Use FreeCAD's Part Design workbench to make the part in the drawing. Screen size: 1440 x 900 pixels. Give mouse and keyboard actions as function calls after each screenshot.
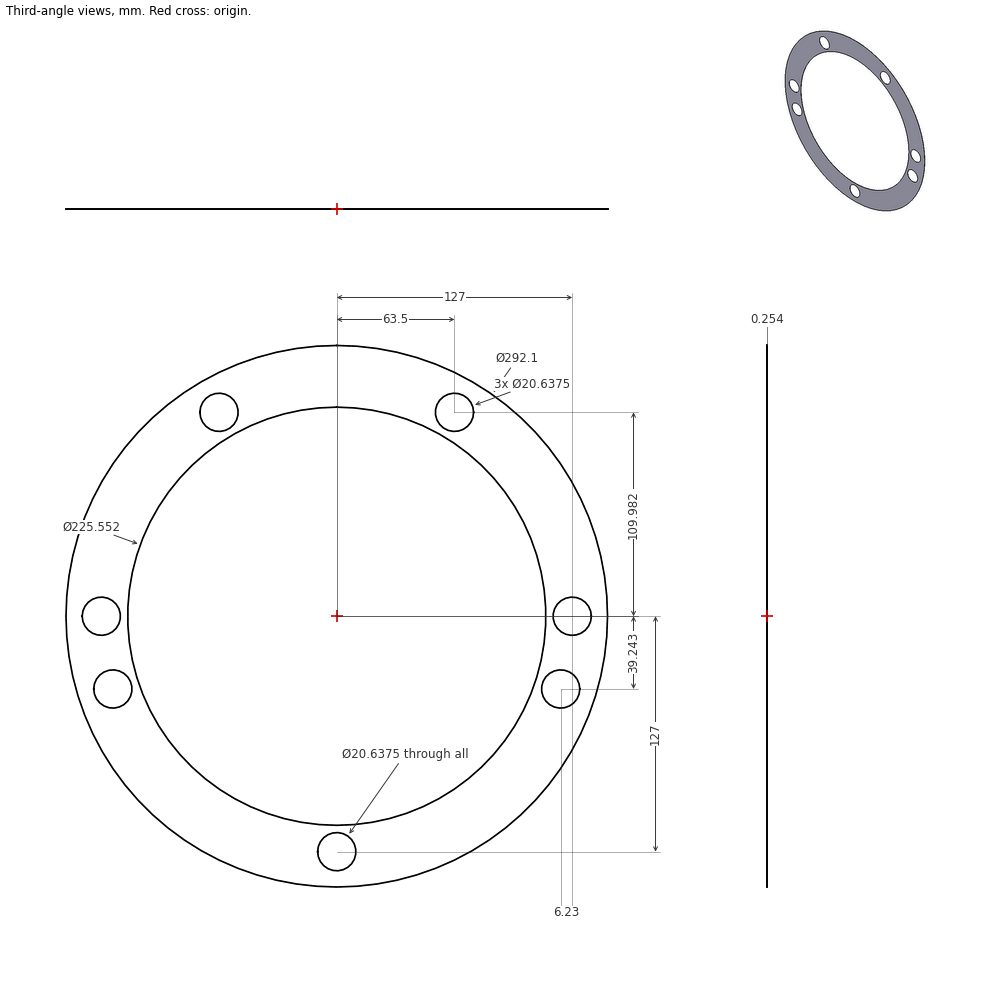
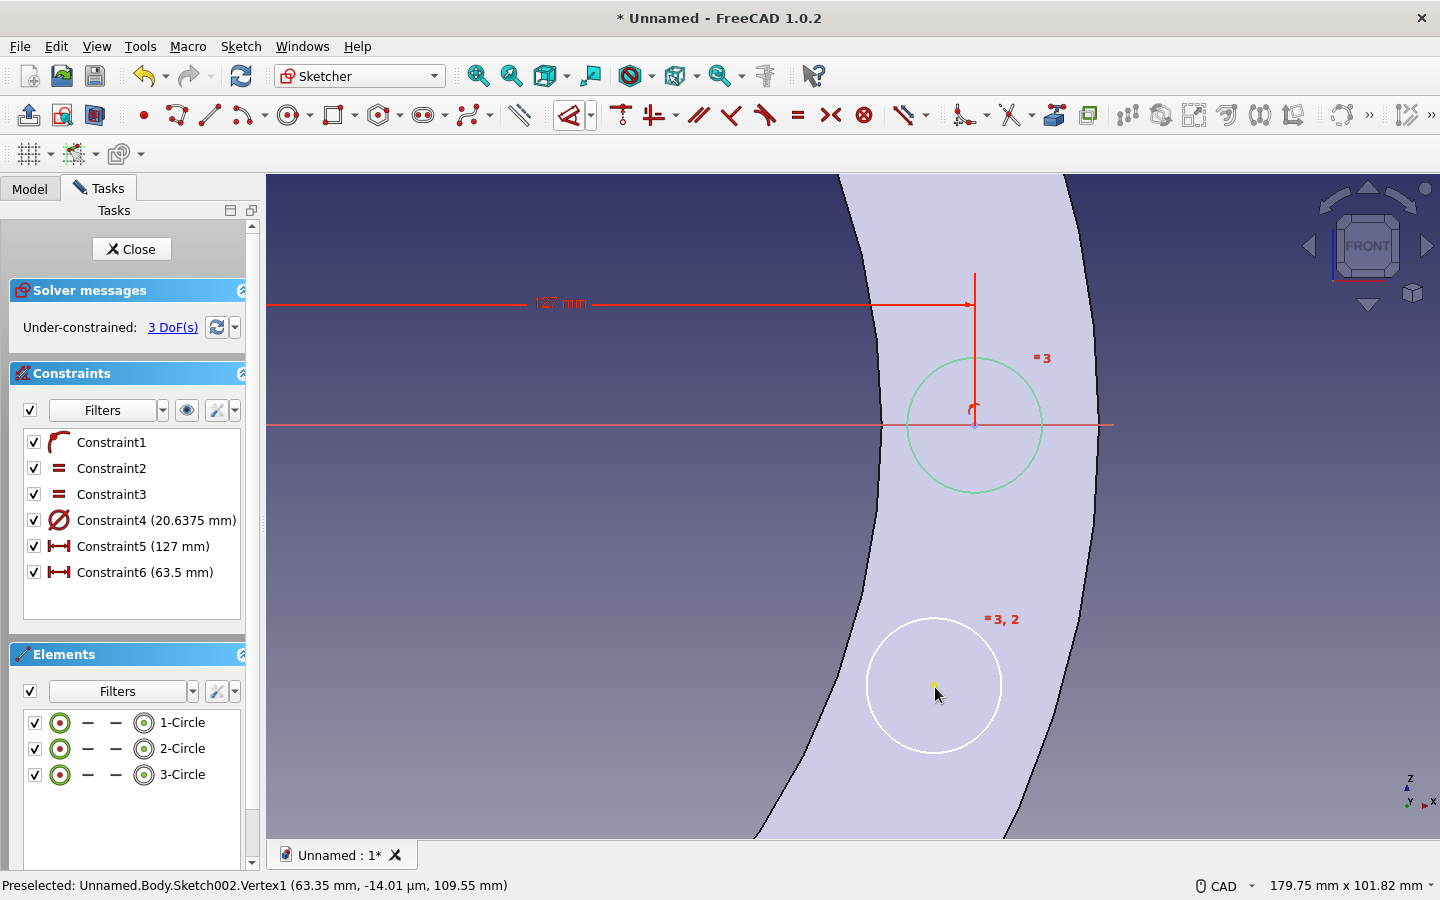
click(934, 686)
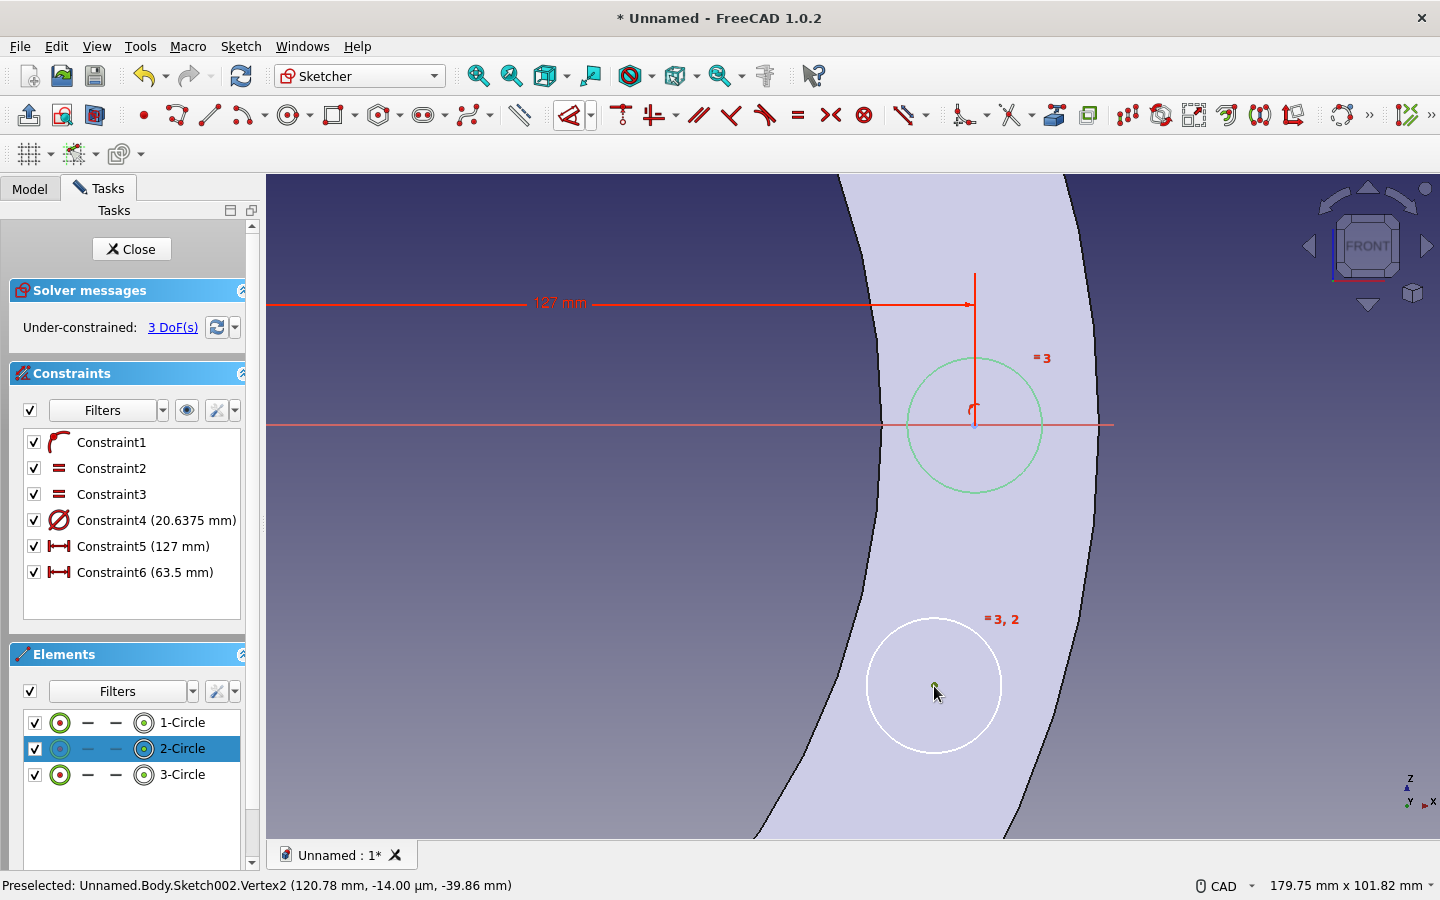
click(975, 425)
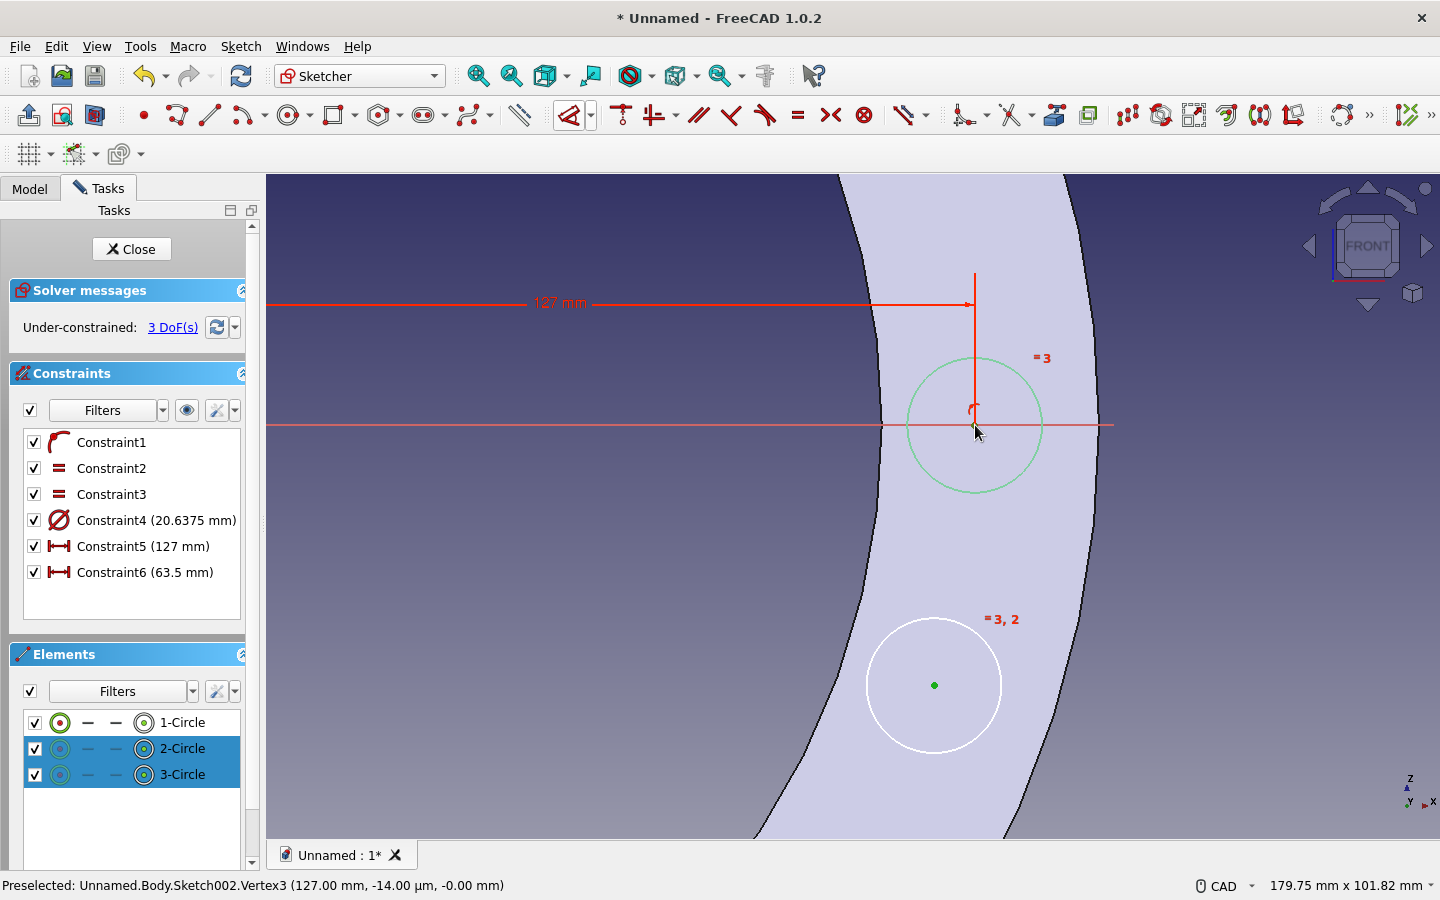
click(590, 116)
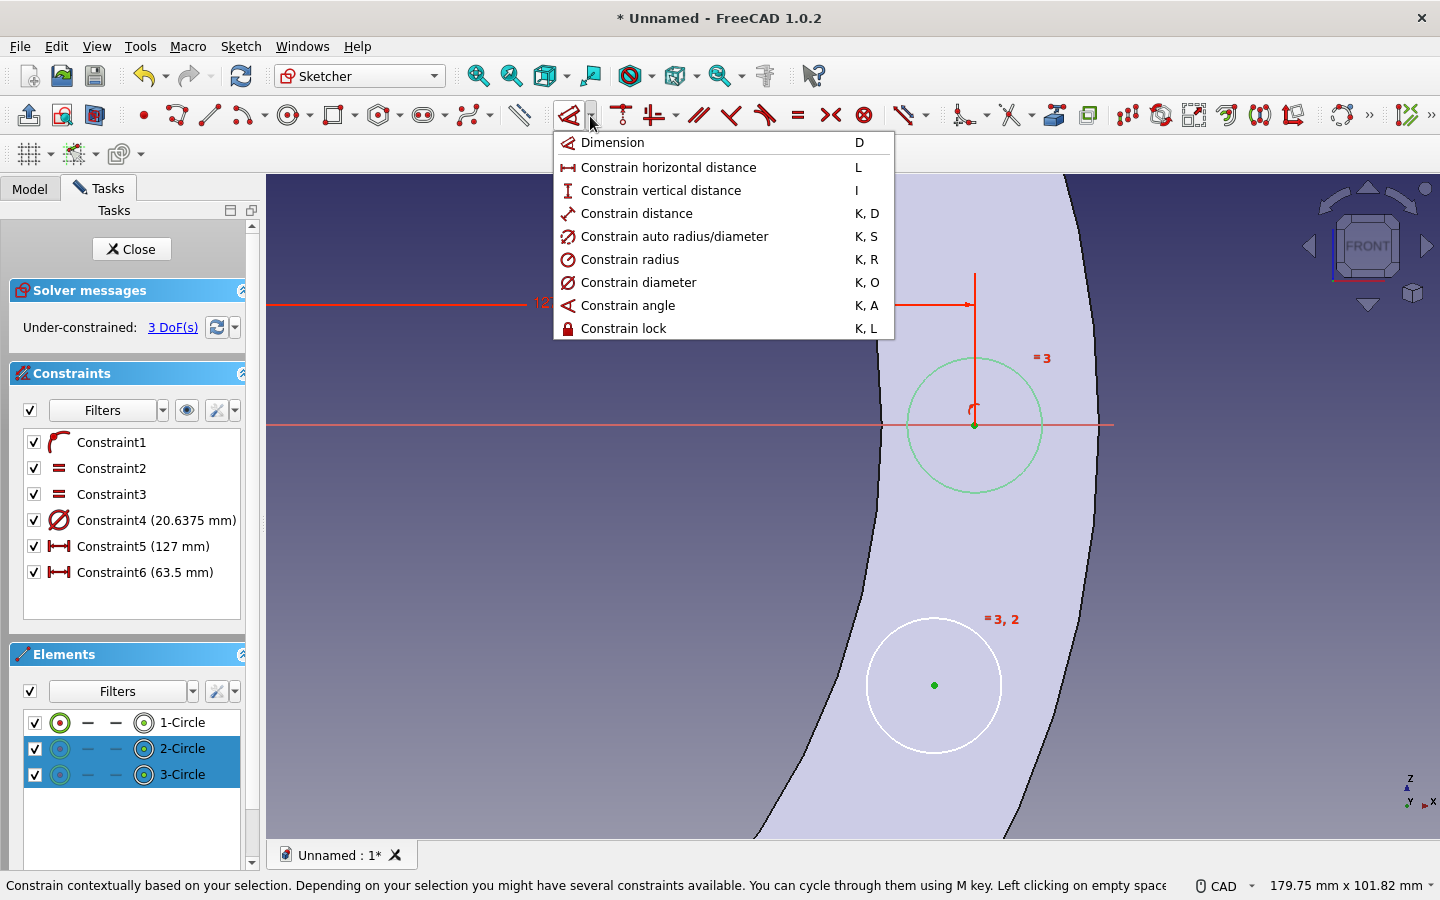
click(724, 168)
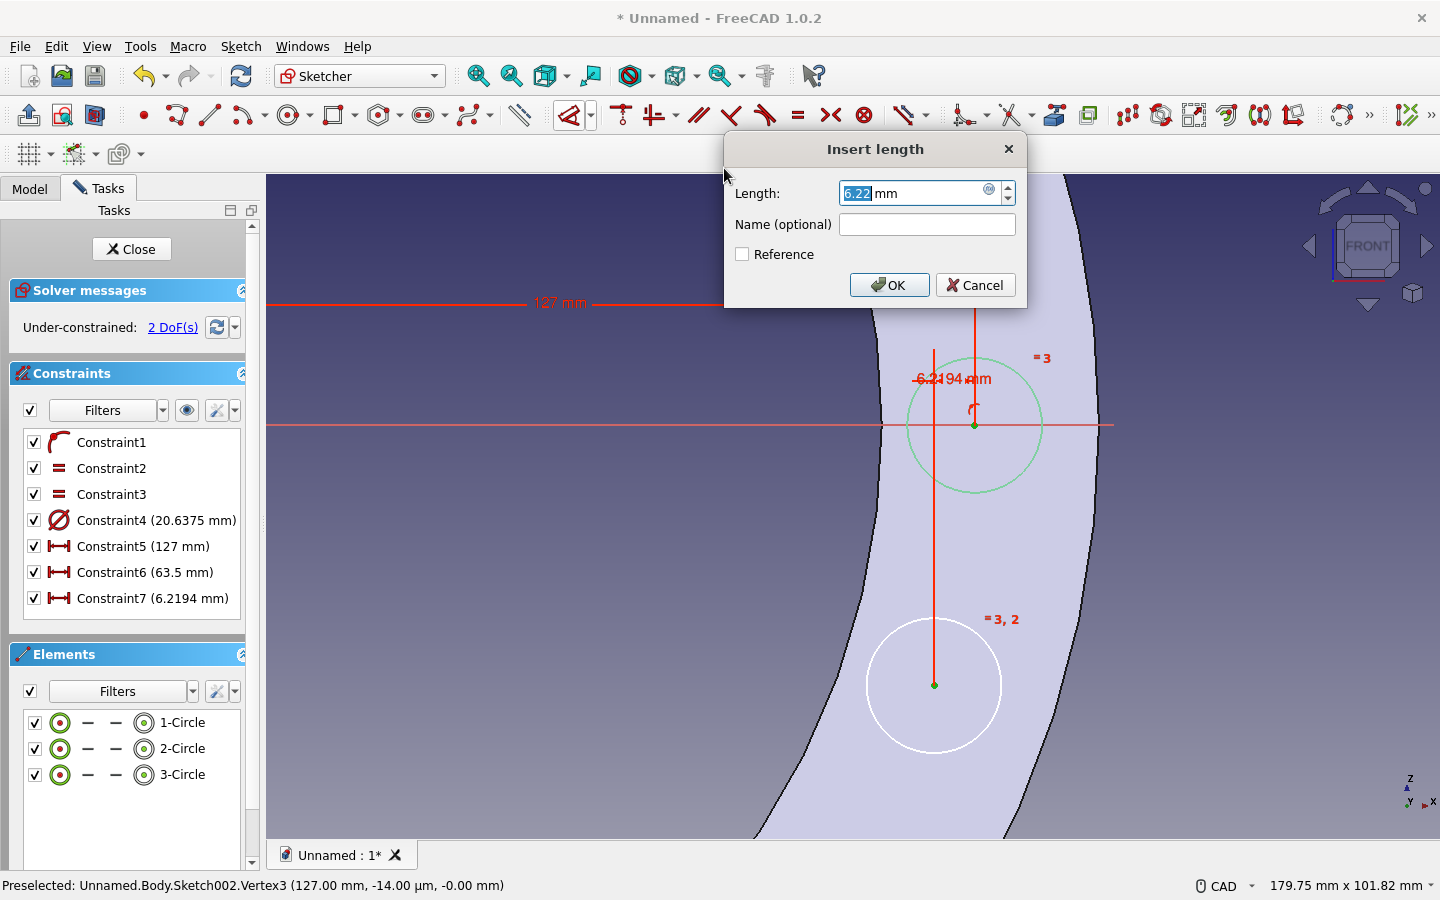
text(6.23)
key(Return)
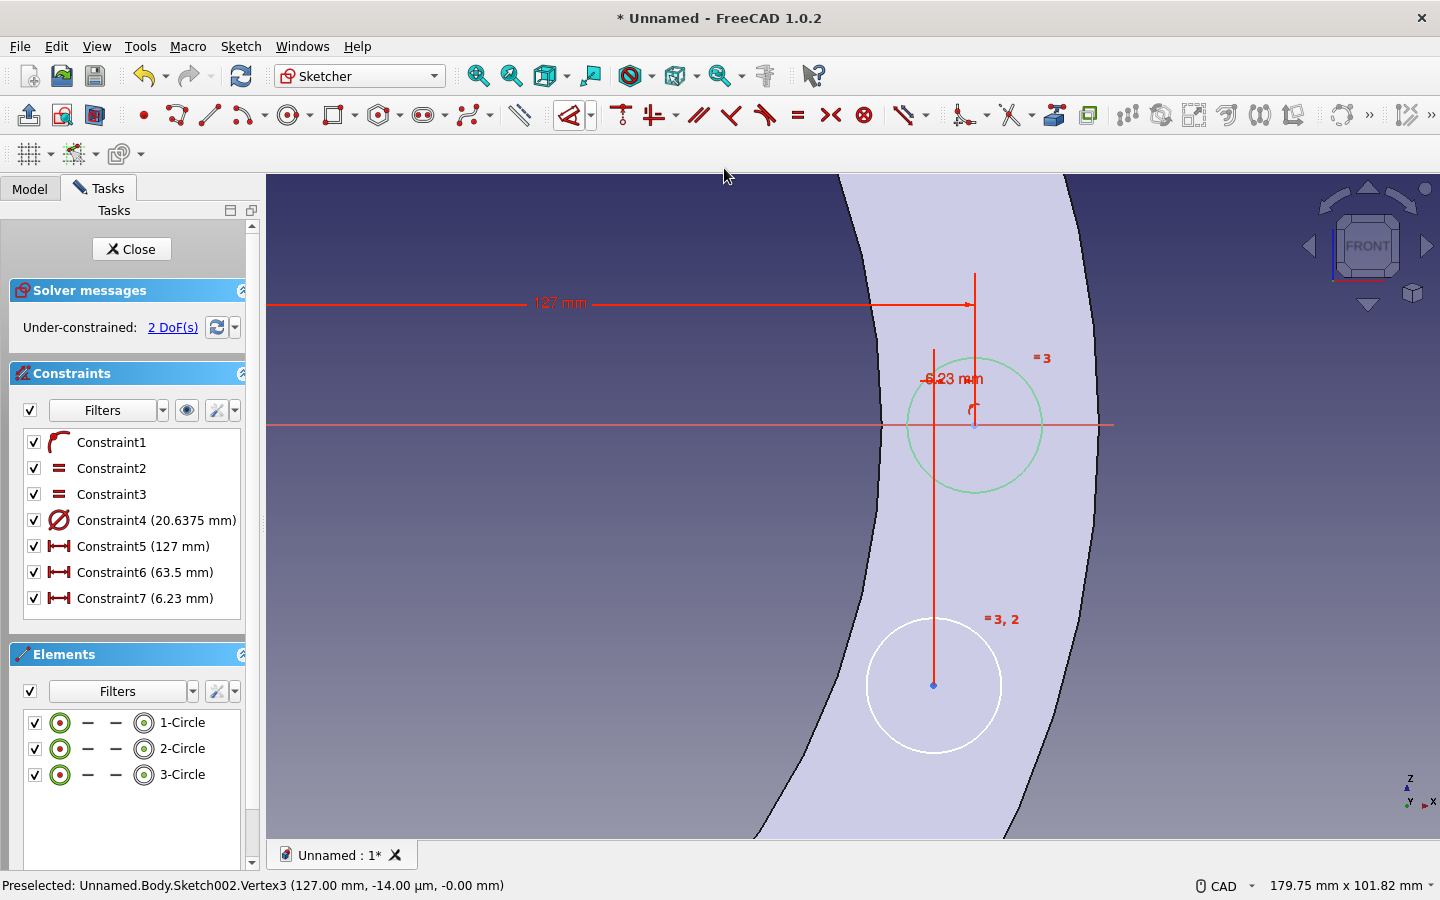
click(934, 686)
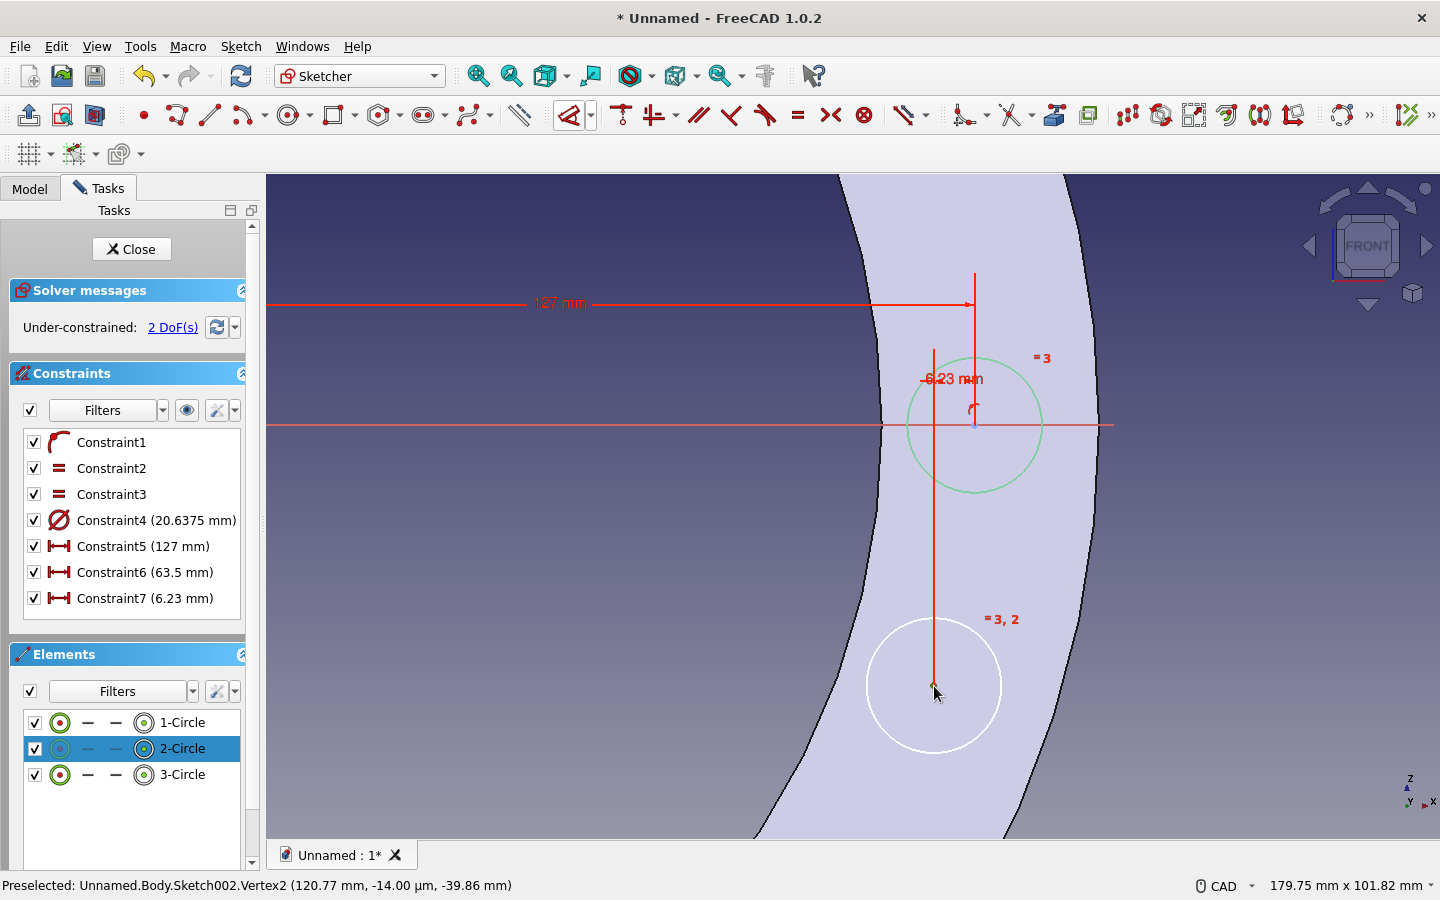
key(i)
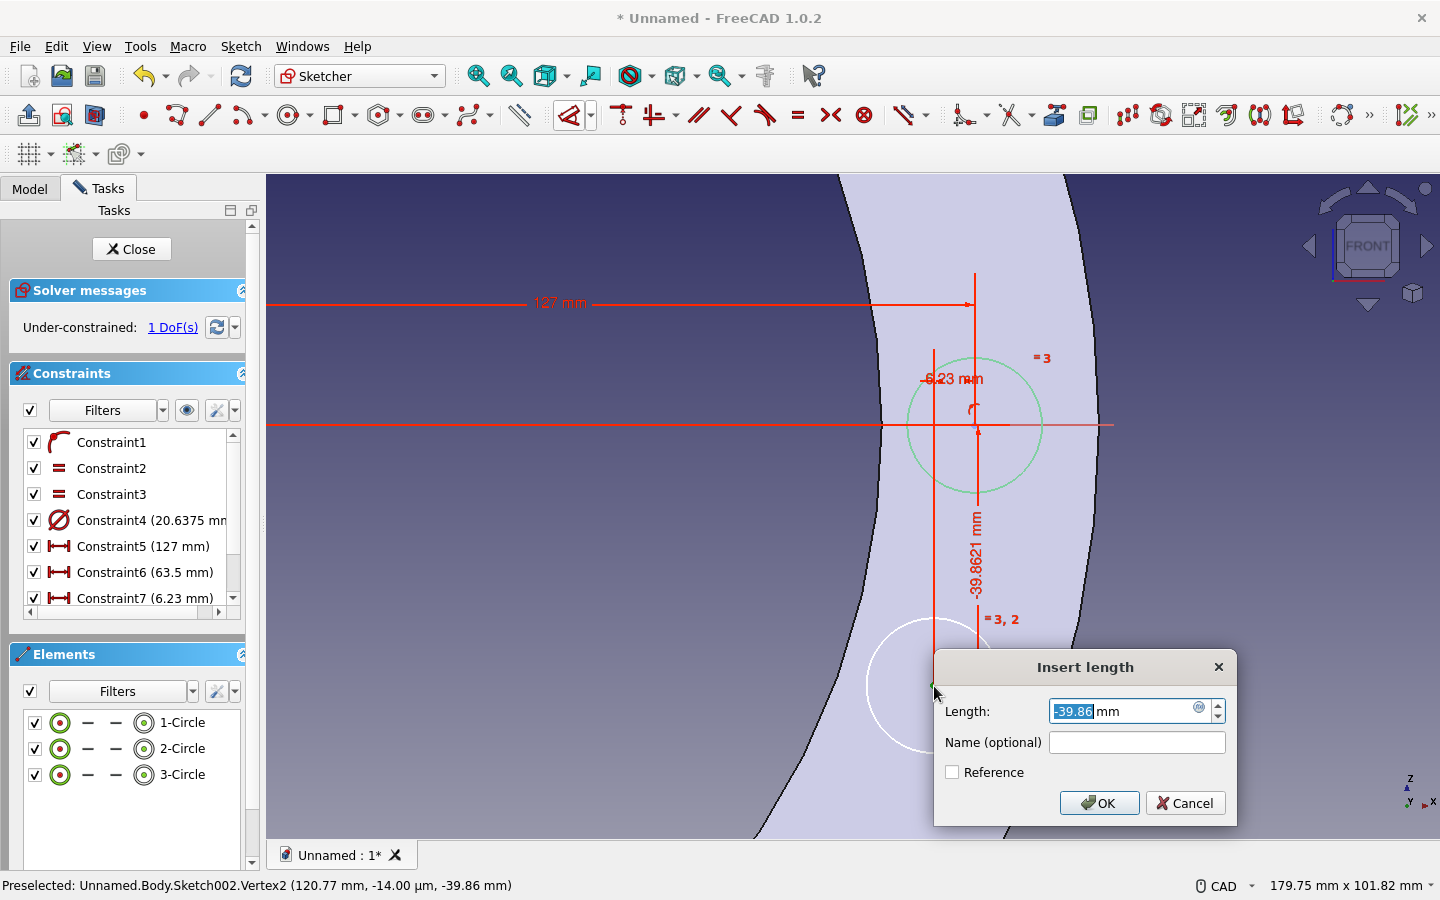
text(-39.243)
key(Return)